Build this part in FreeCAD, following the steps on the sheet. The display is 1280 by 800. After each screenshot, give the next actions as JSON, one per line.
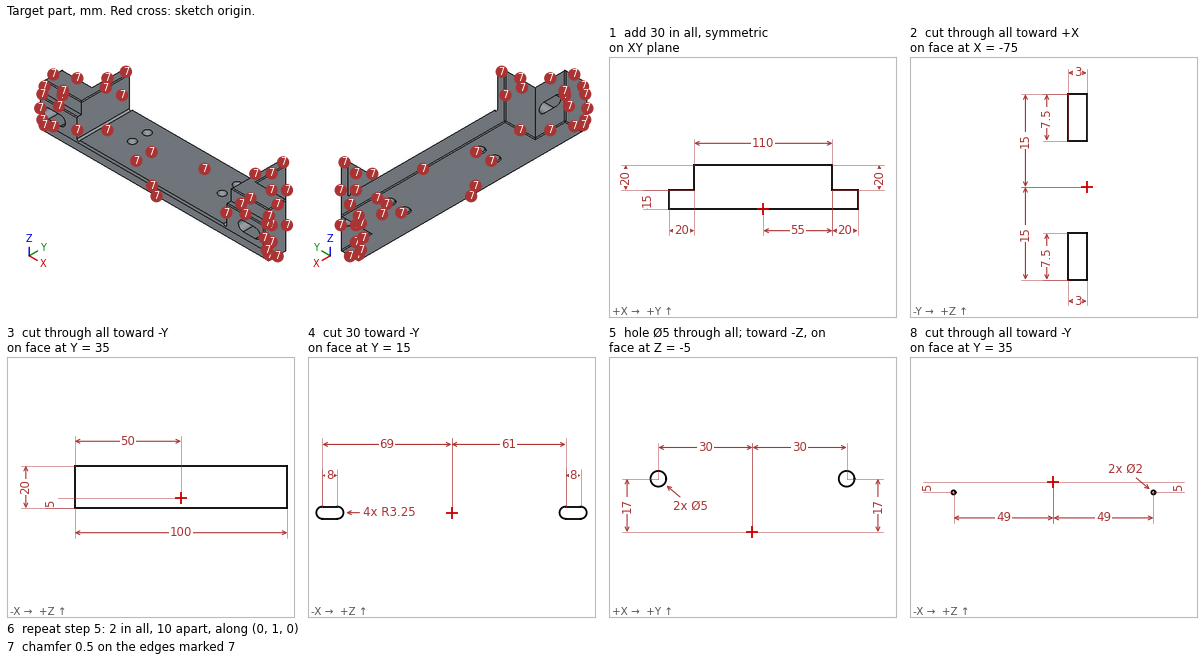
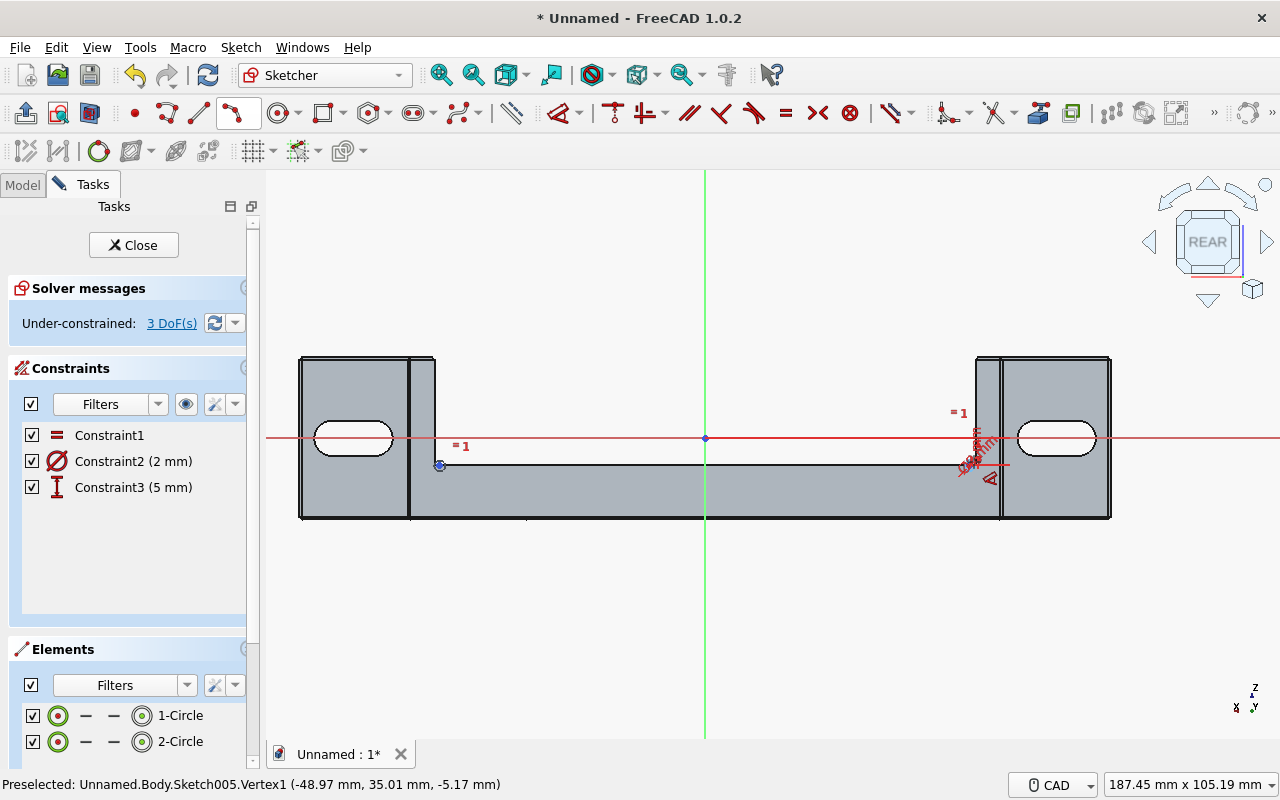
{"action": "scroll", "coordinate": [440, 466], "scroll_direction": "up", "scroll_amount": 2}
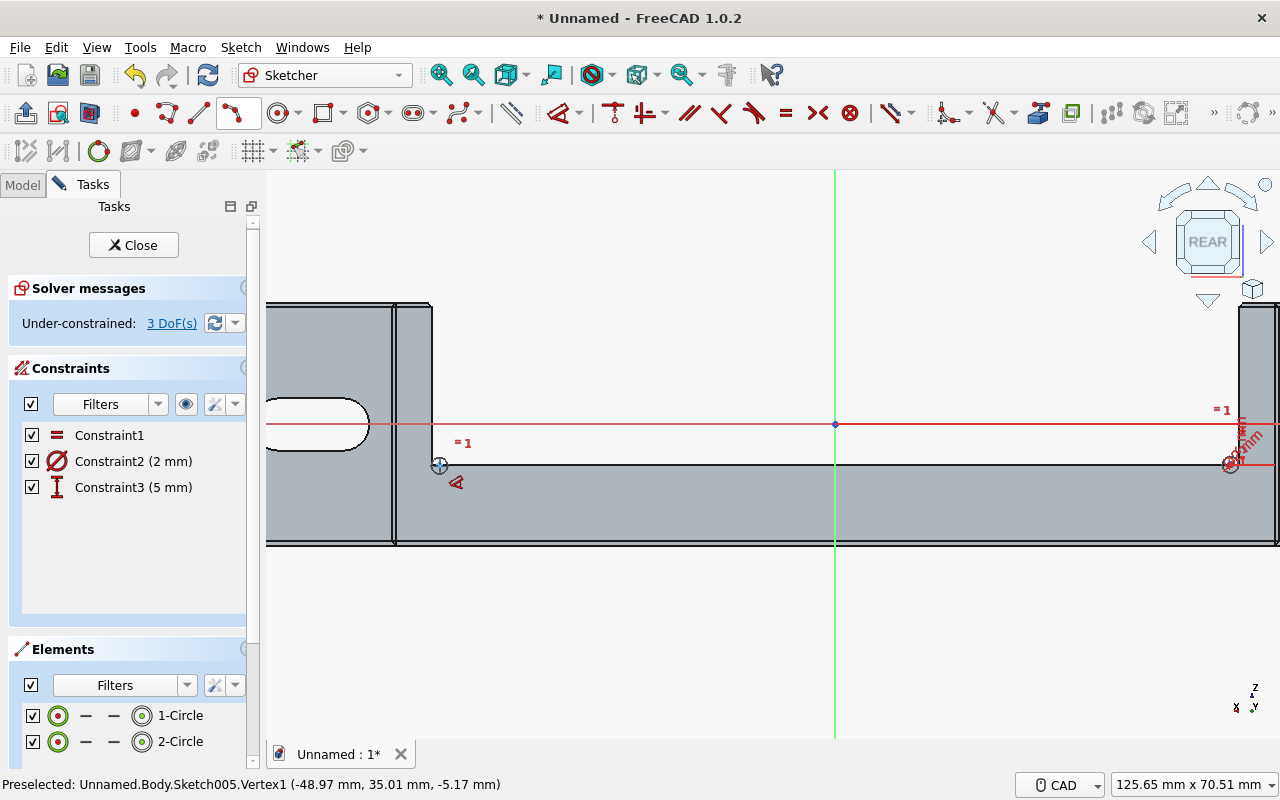
{"action": "left_click", "coordinate": [440, 466]}
{"action": "left_click", "coordinate": [406, 445]}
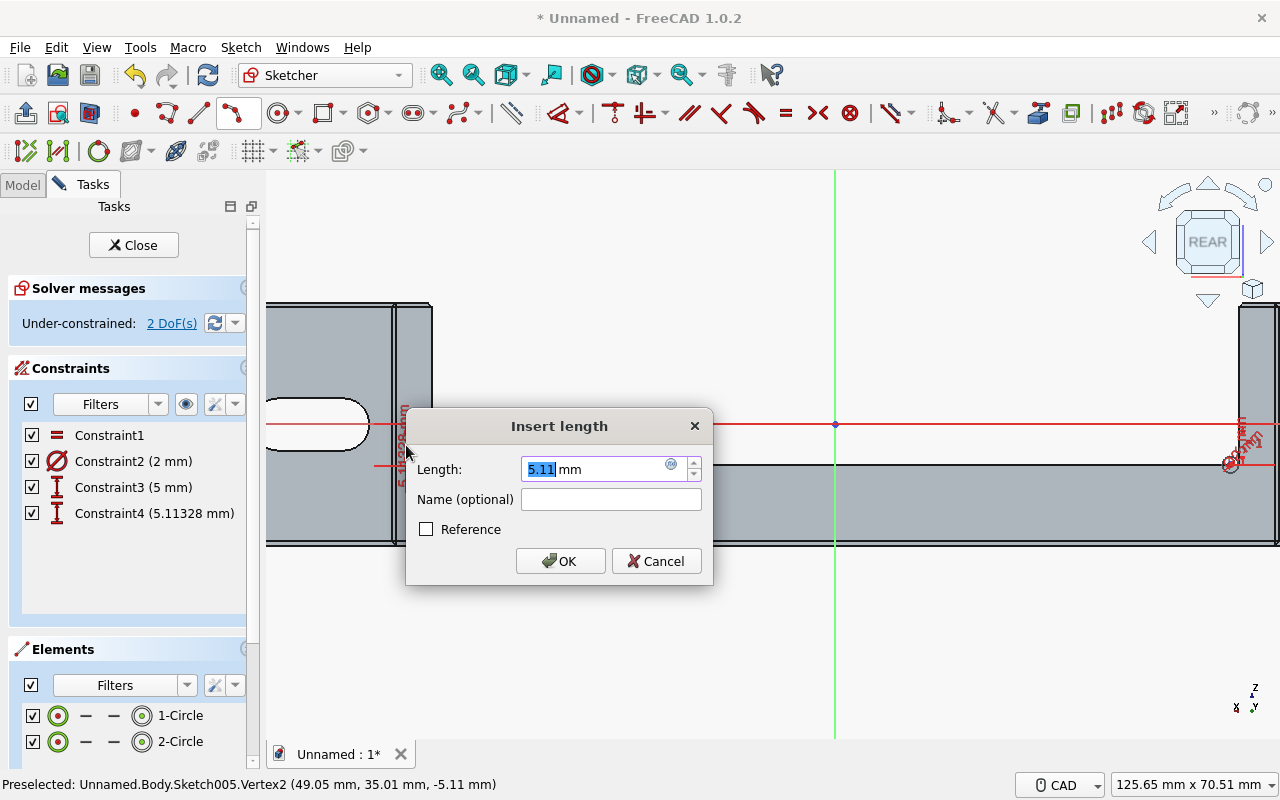
{"action": "type", "text": "5"}
{"action": "key", "text": "Return"}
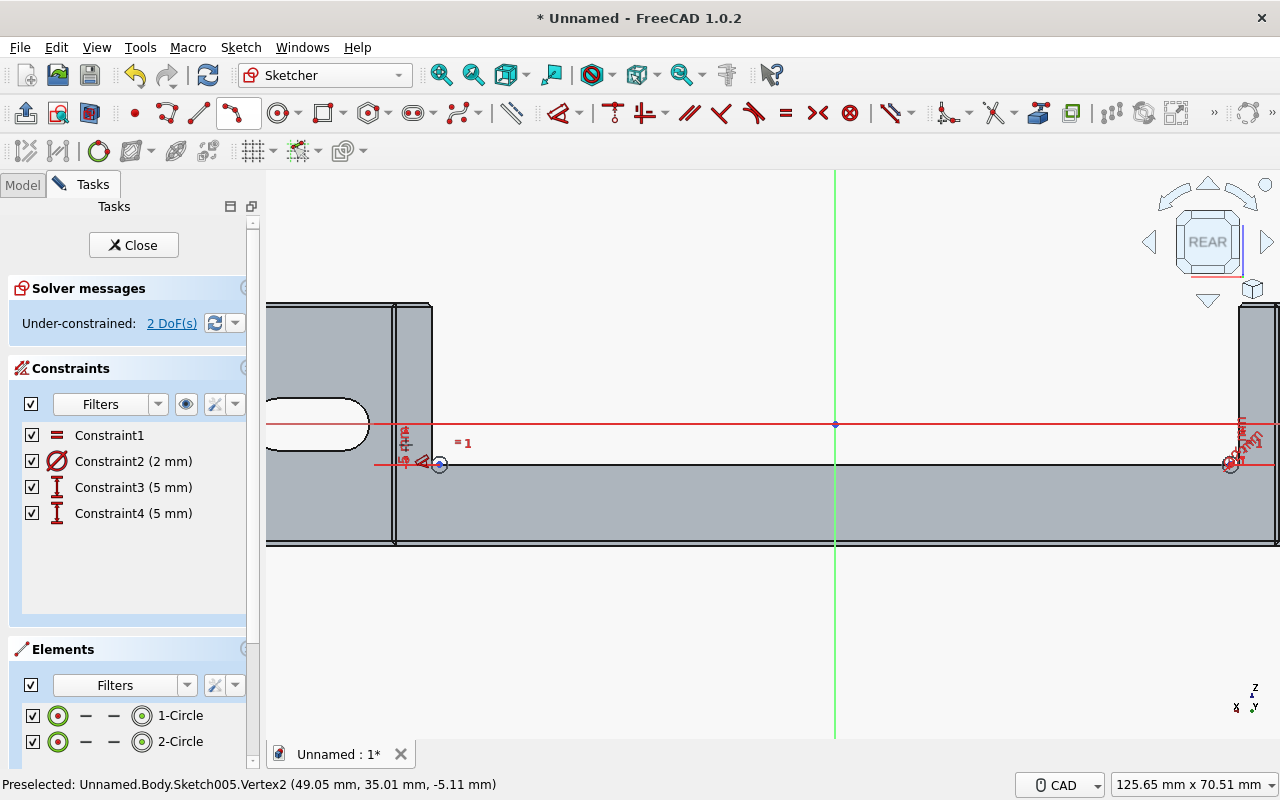
{"action": "scroll", "coordinate": [438, 466], "scroll_direction": "down", "scroll_amount": 2}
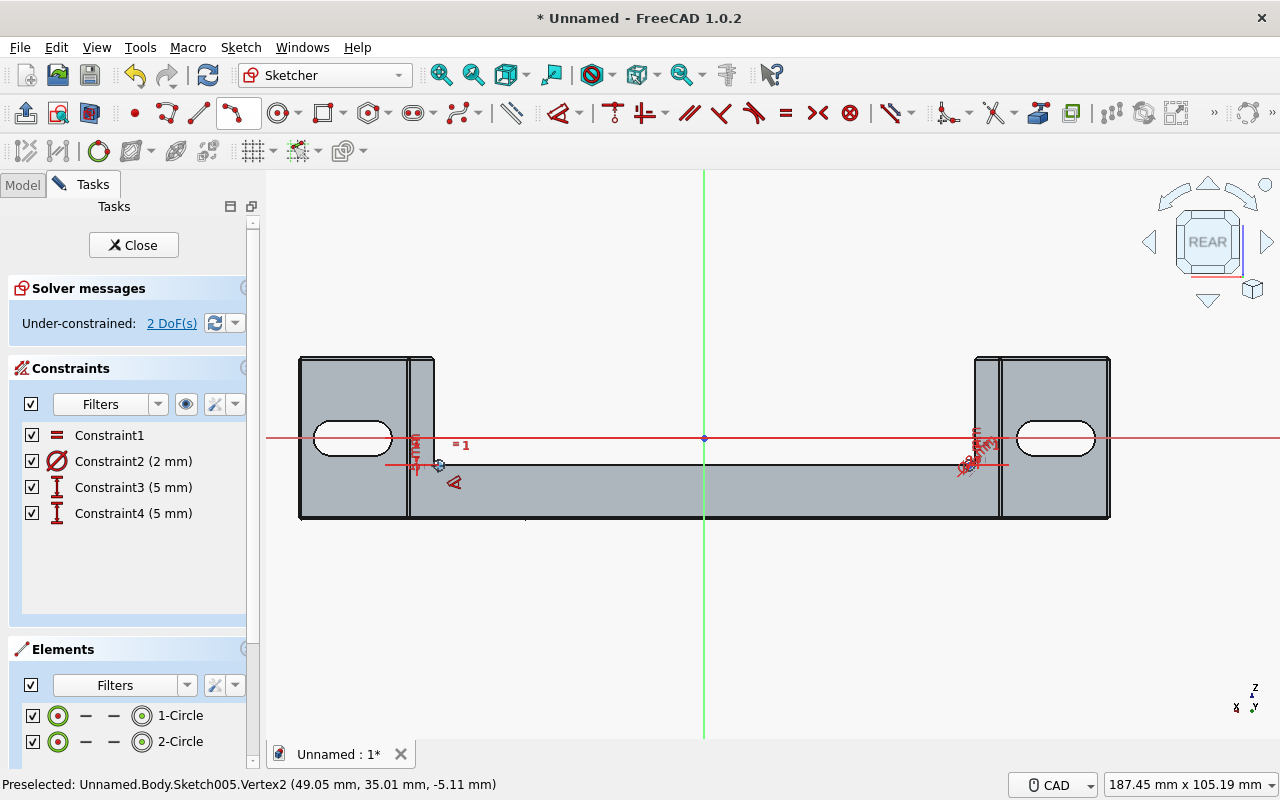
{"action": "left_click", "coordinate": [969, 465]}
{"action": "left_click", "coordinate": [837, 404]}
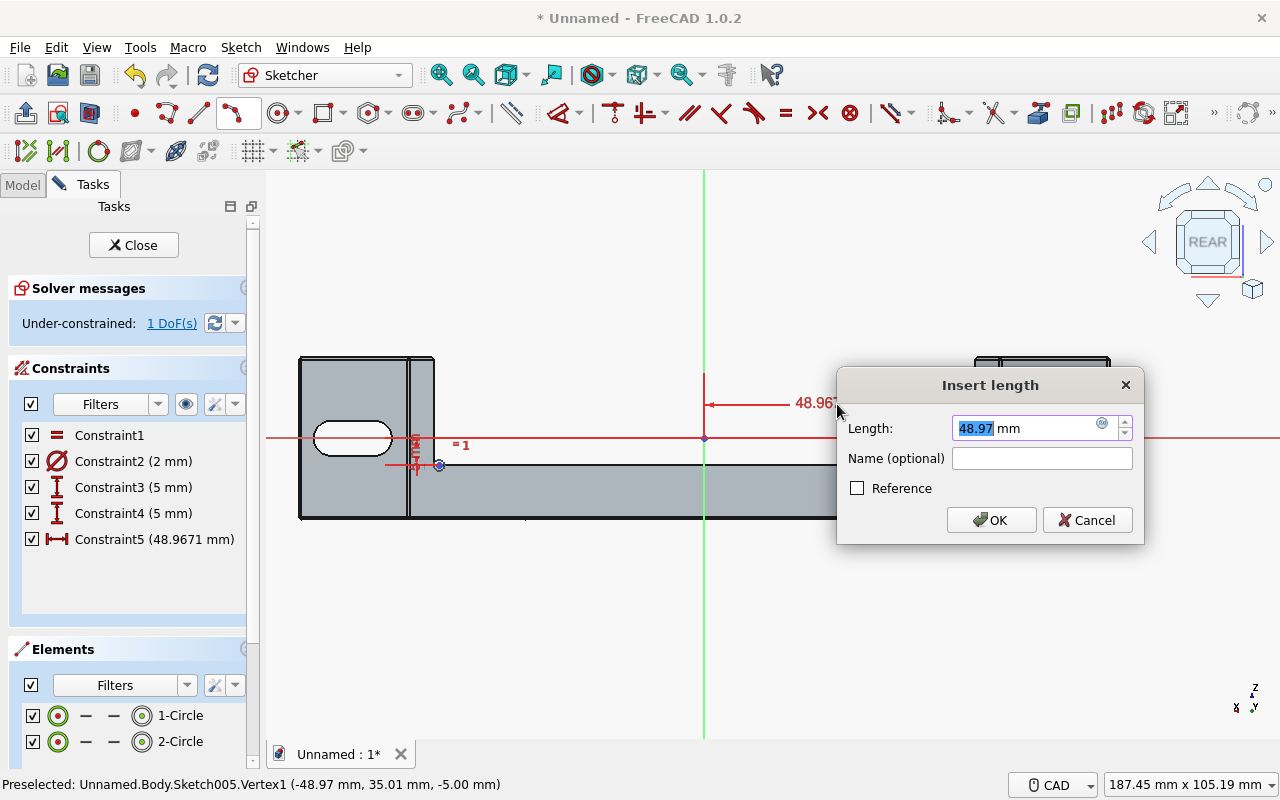
{"action": "type", "text": "49"}
{"action": "key", "text": "Return"}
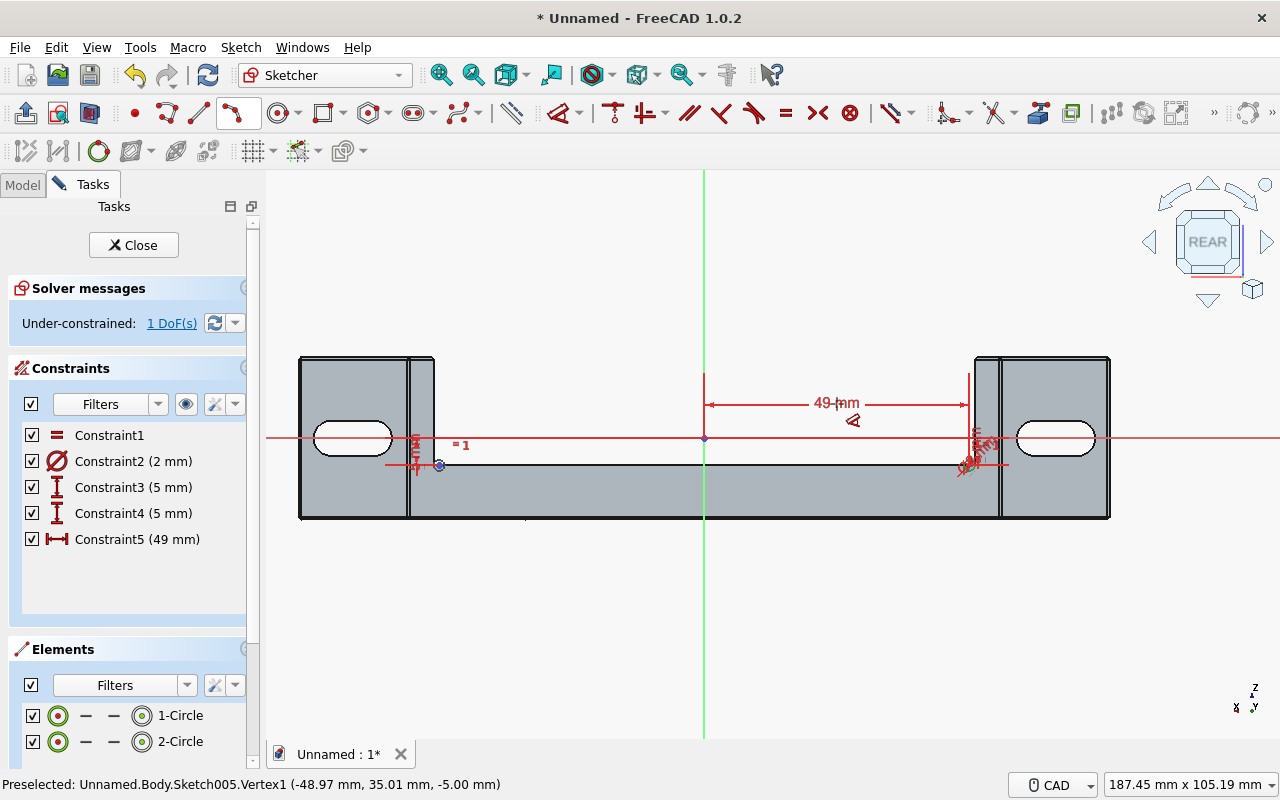
{"action": "left_click", "coordinate": [439, 465]}
{"action": "left_click", "coordinate": [572, 404]}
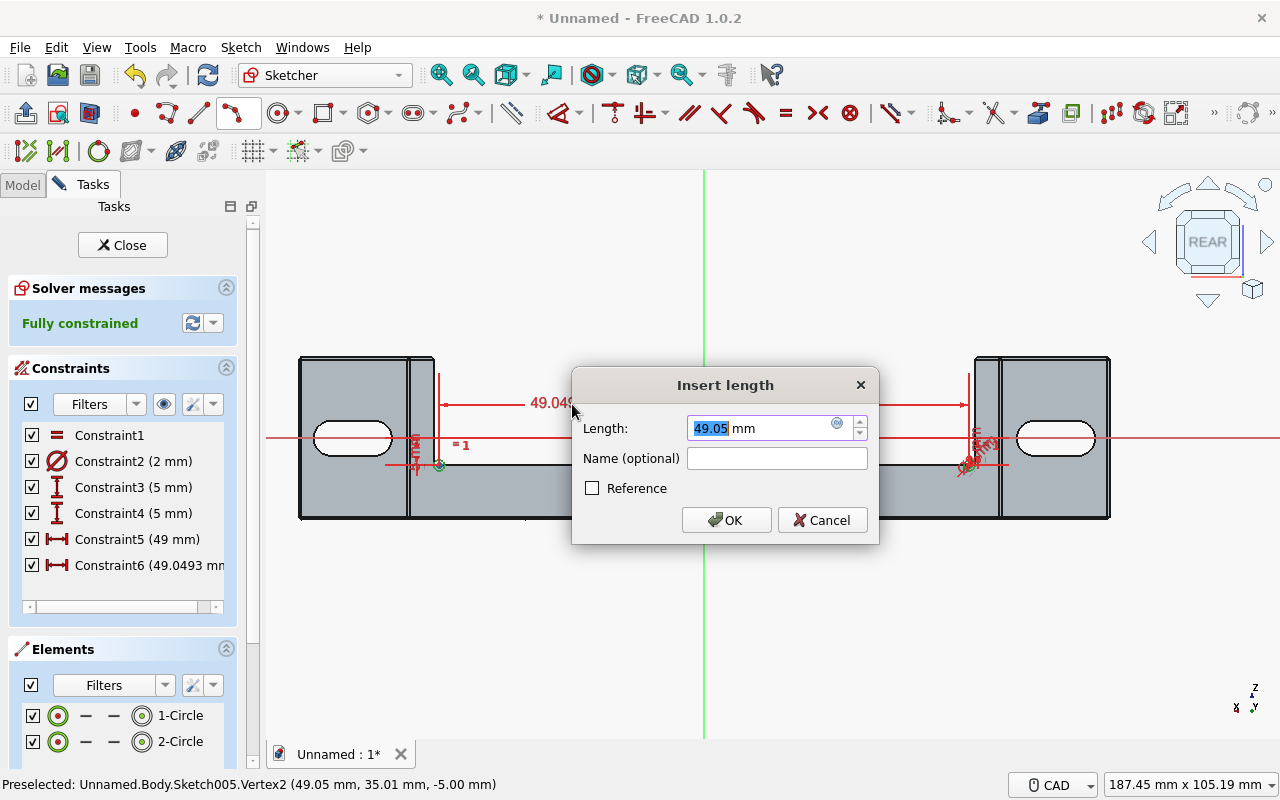
{"action": "type", "text": "49"}
{"action": "key", "text": "Return"}
{"action": "key", "text": "Escape"}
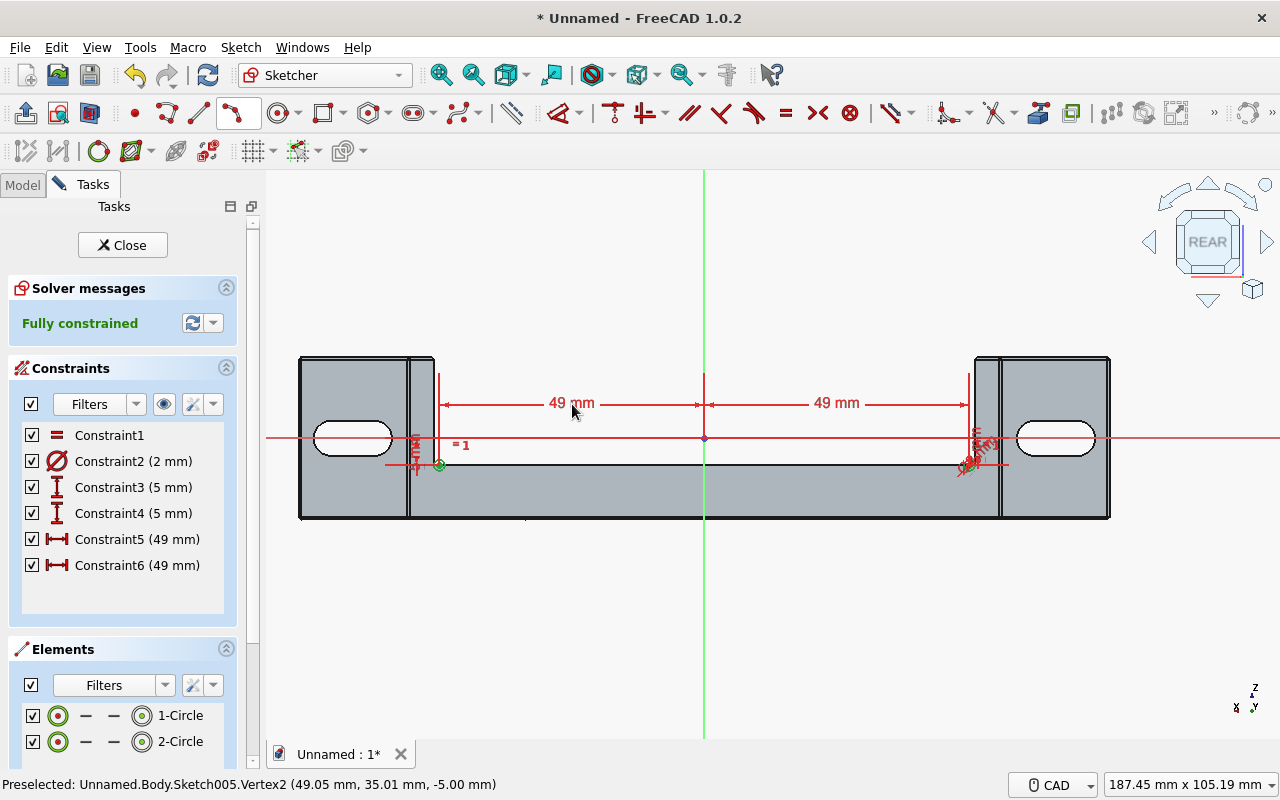
{"action": "left_click", "coordinate": [123, 245]}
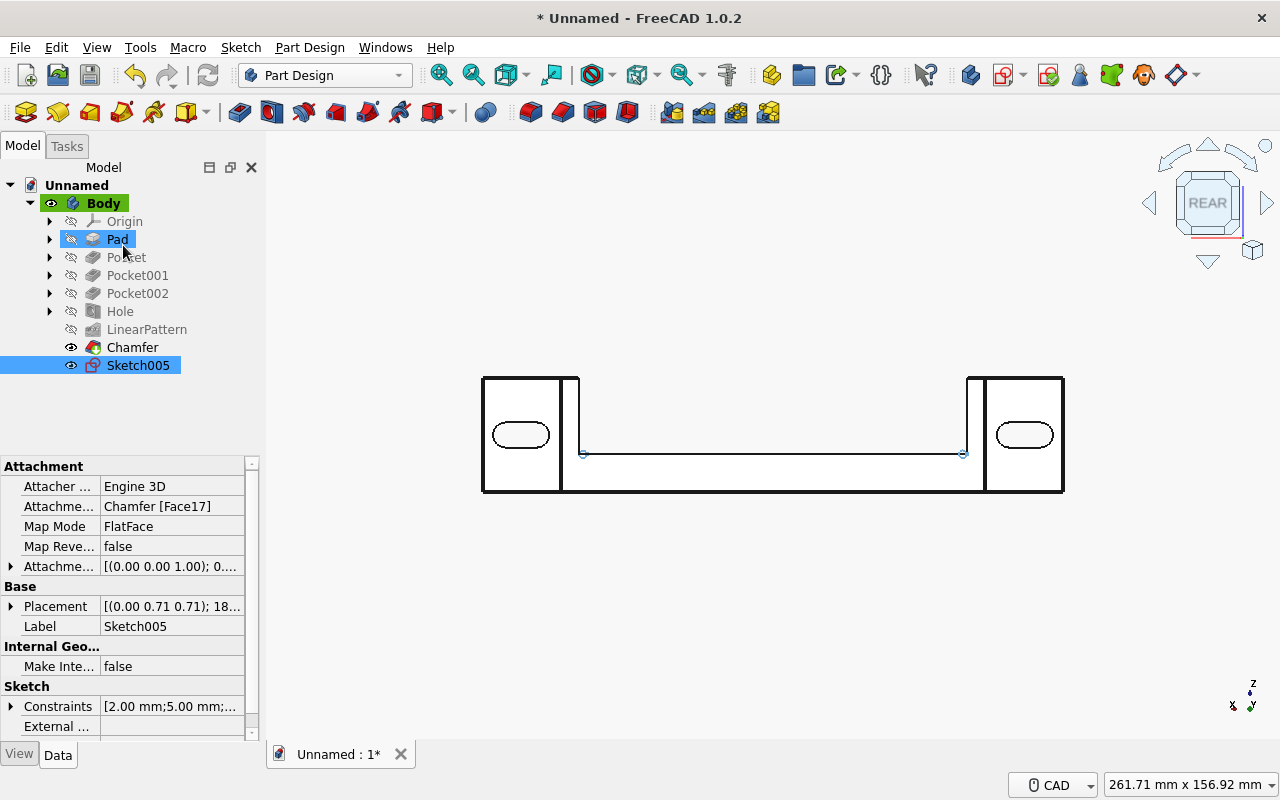
{"action": "left_click", "coordinate": [240, 112]}